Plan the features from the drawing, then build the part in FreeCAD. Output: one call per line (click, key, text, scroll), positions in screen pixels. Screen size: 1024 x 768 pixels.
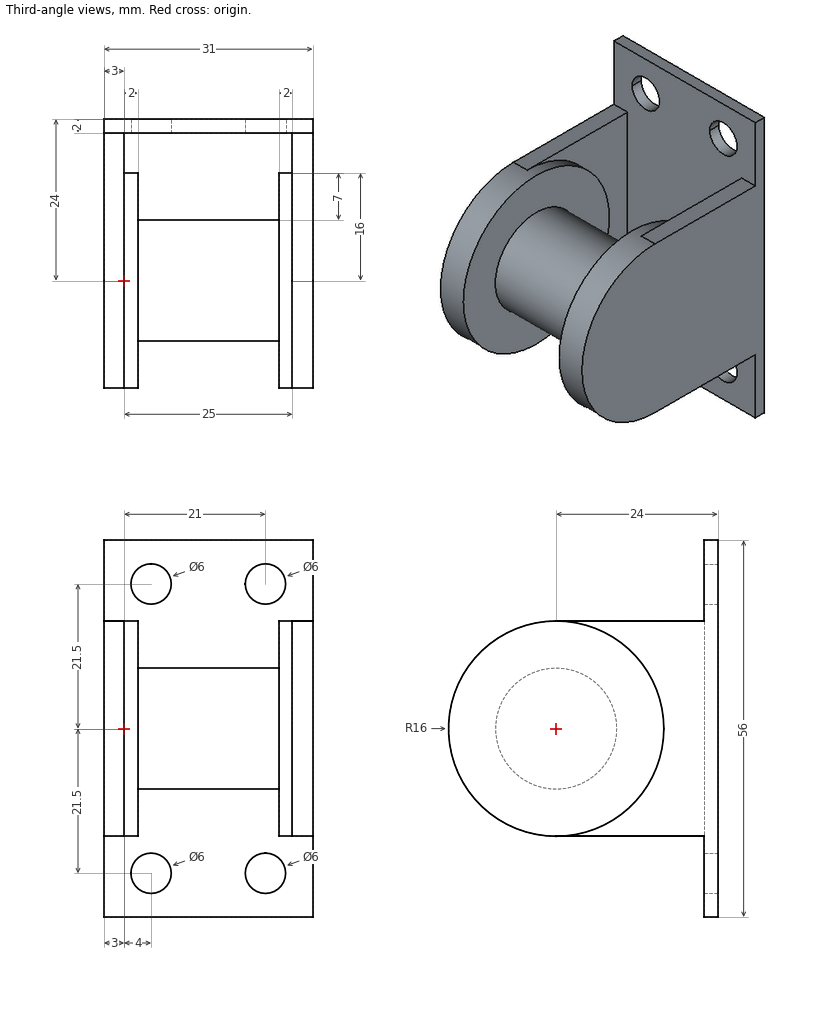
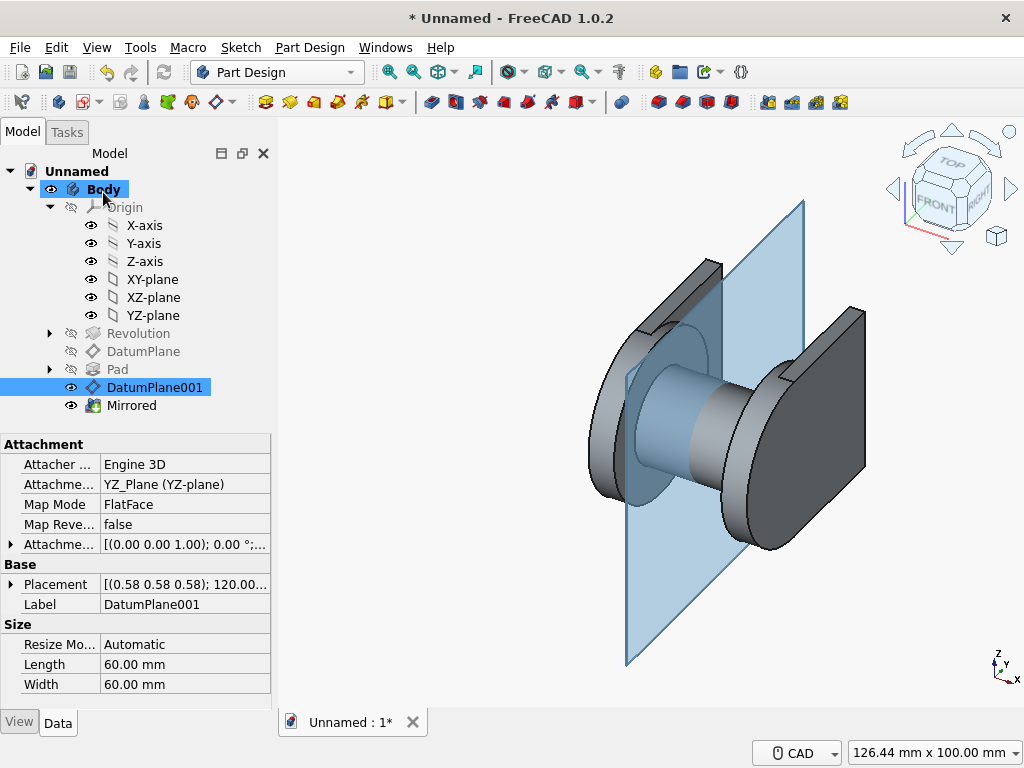
click(116, 387)
key(space)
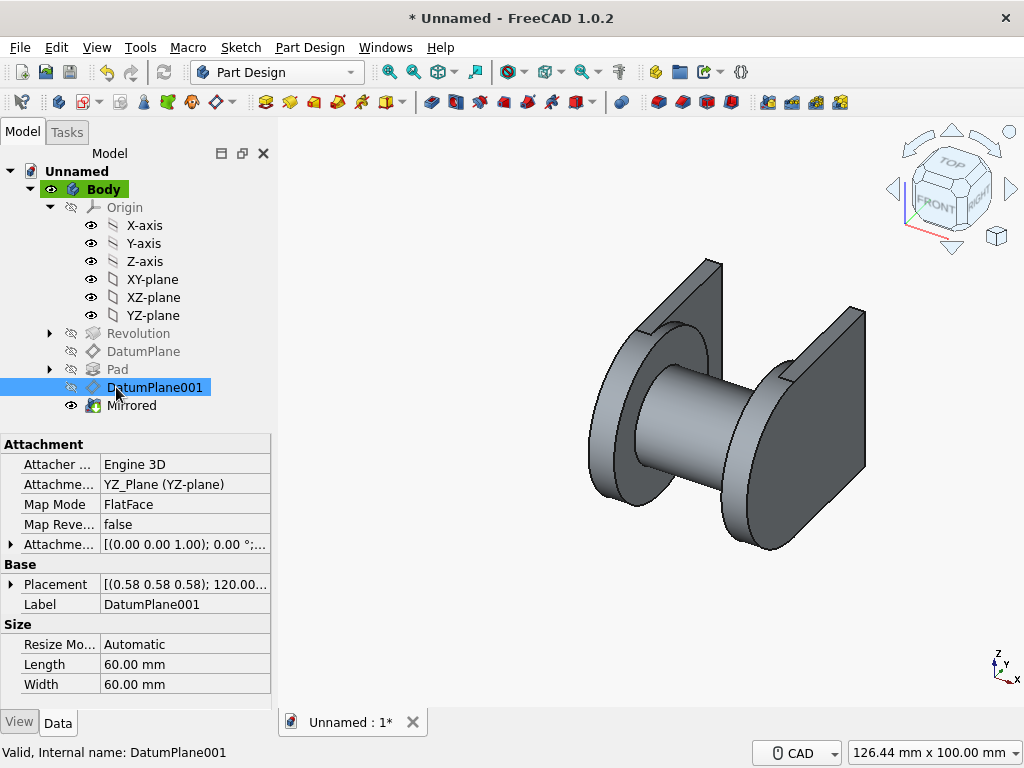
click(318, 667)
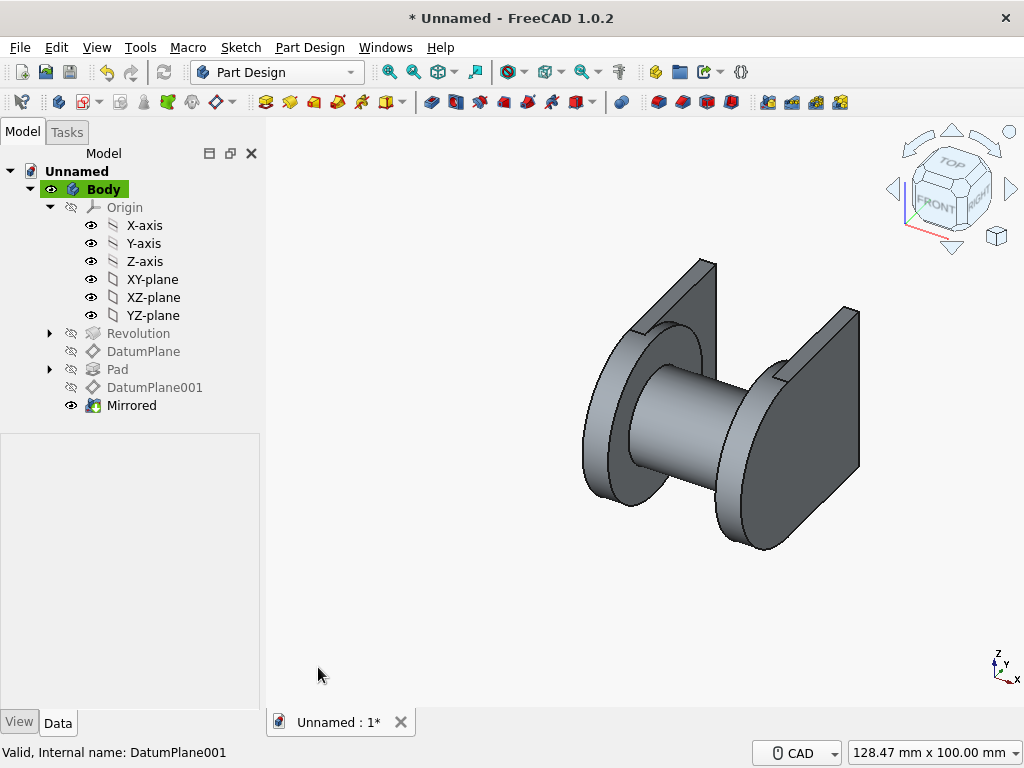
click(84, 102)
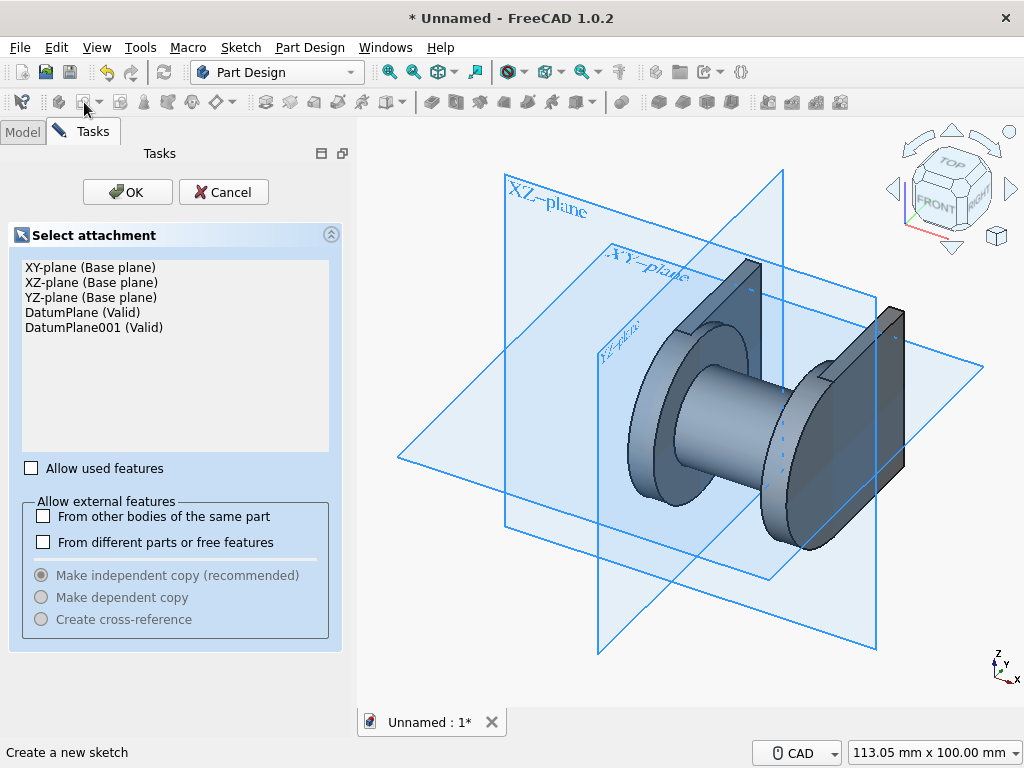
click(82, 268)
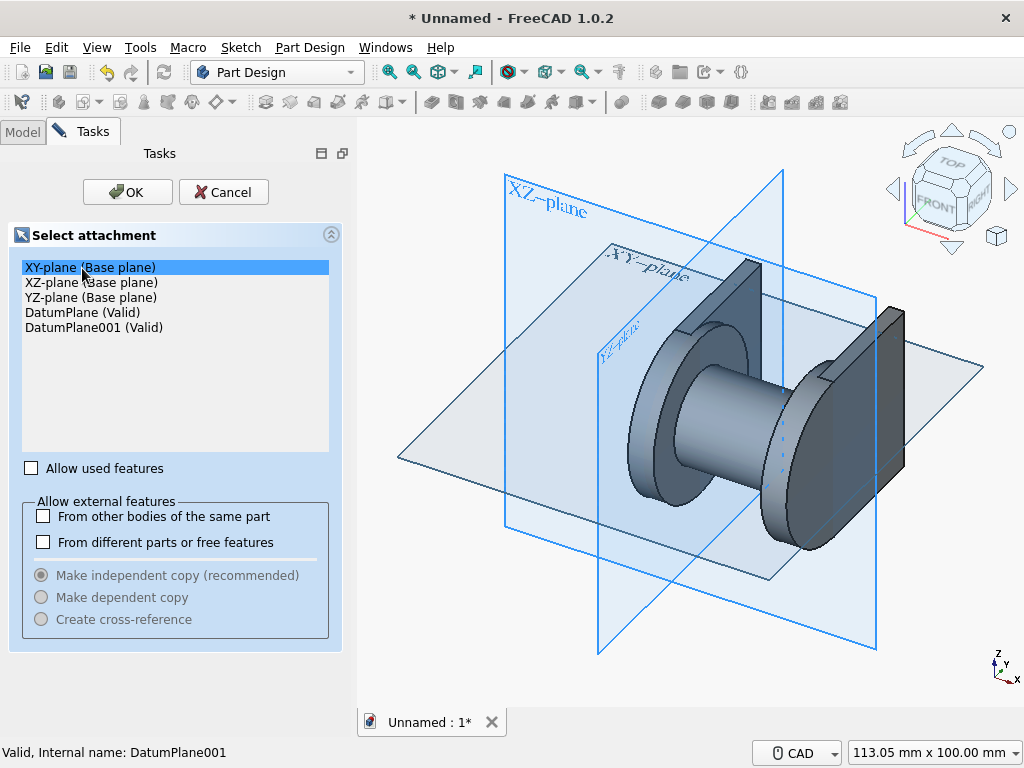
click(128, 192)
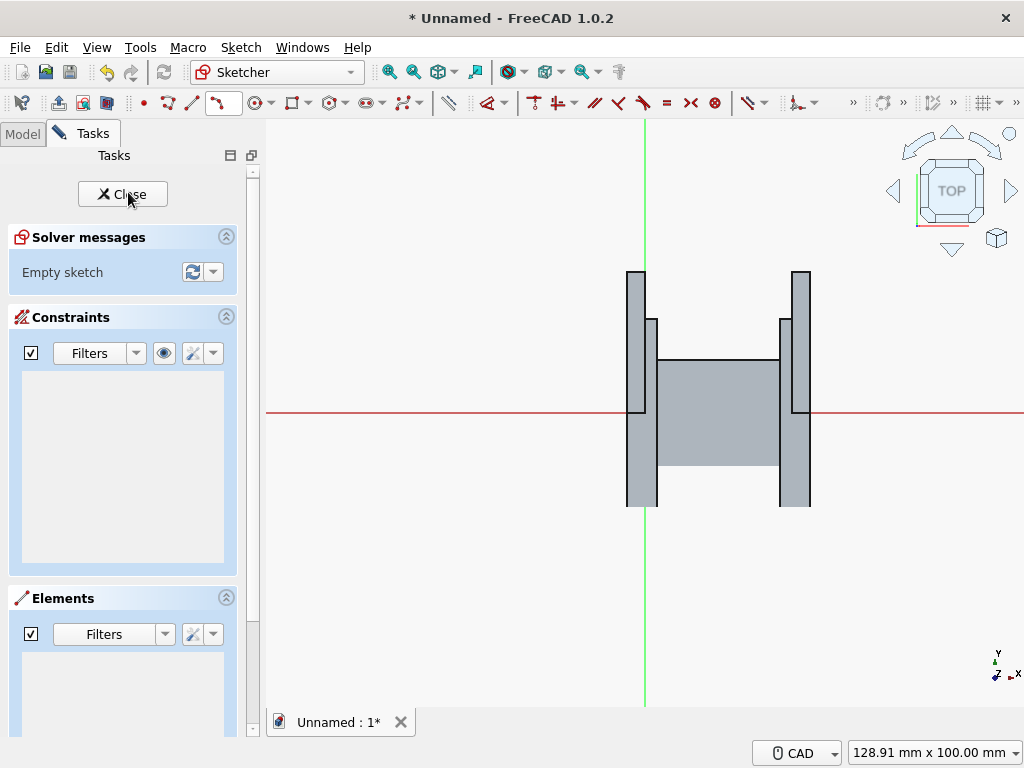
click(108, 104)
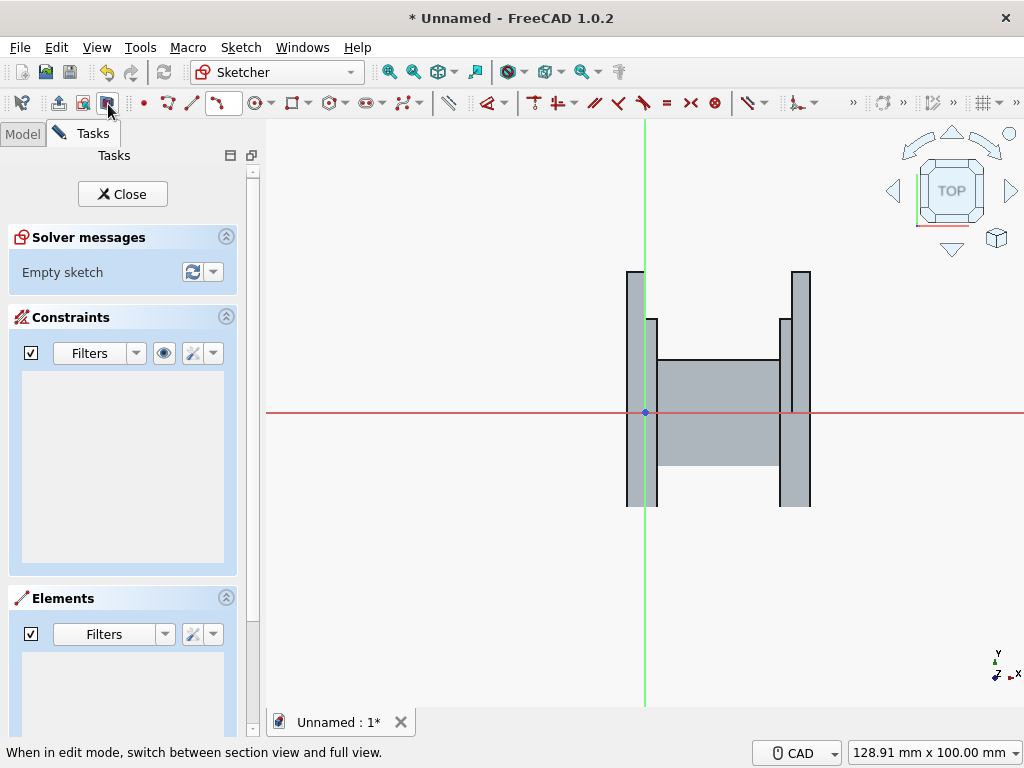
scroll(834, 285, up, 4)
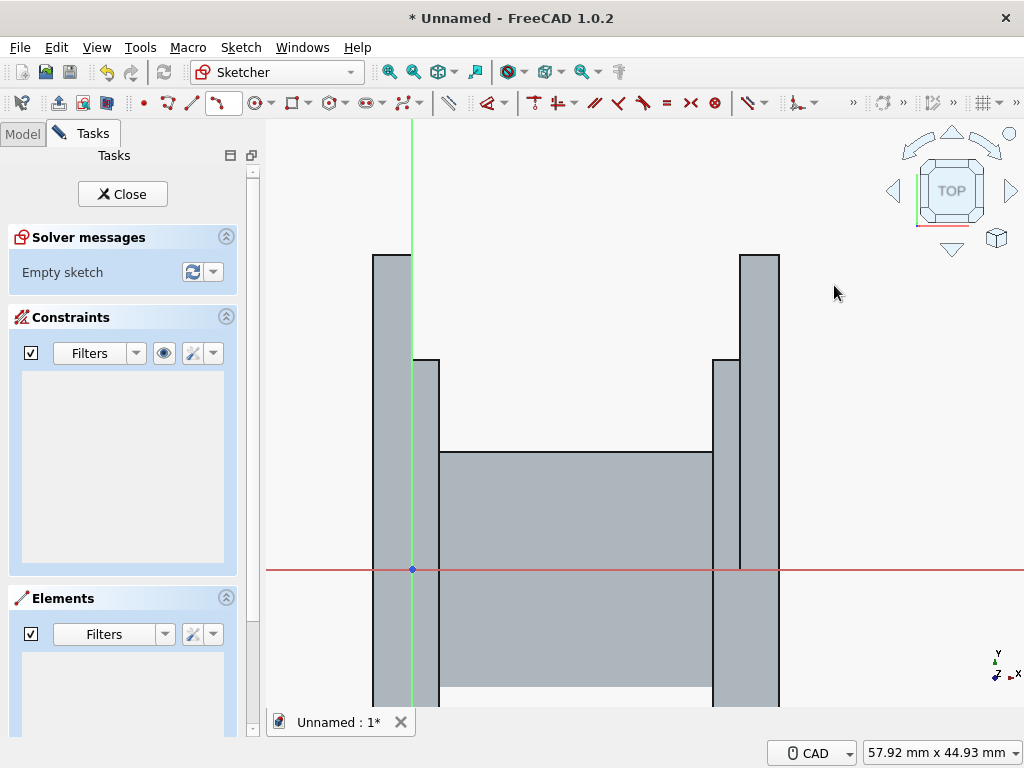
click(292, 104)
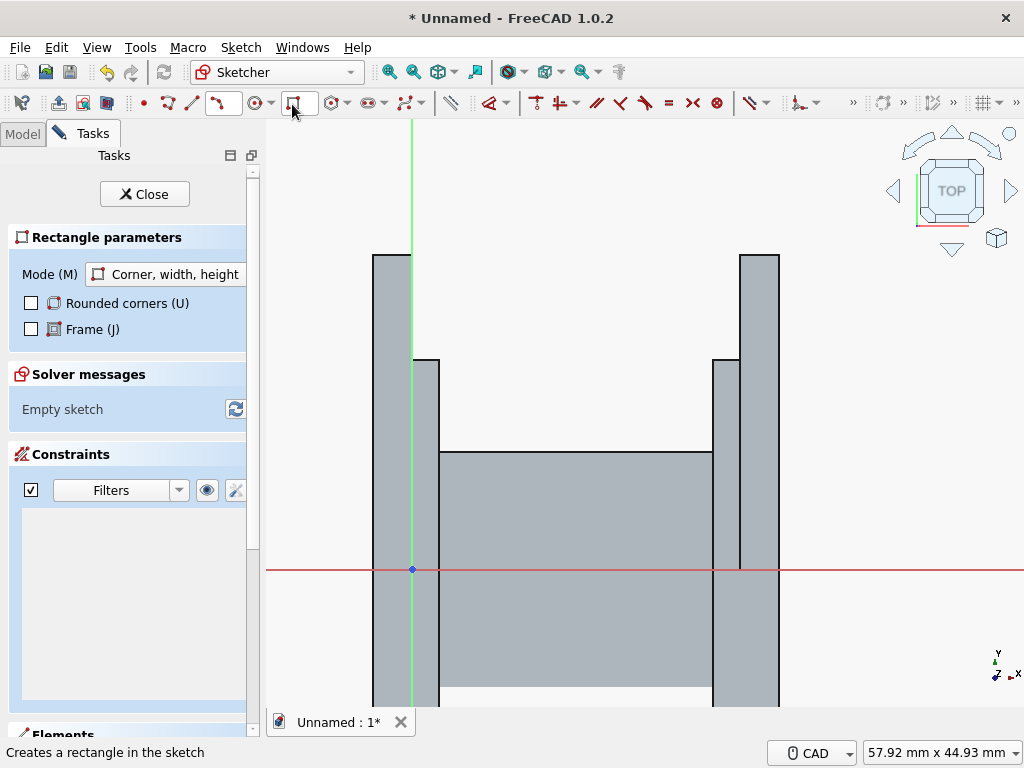
click(373, 255)
click(779, 282)
key(Escape)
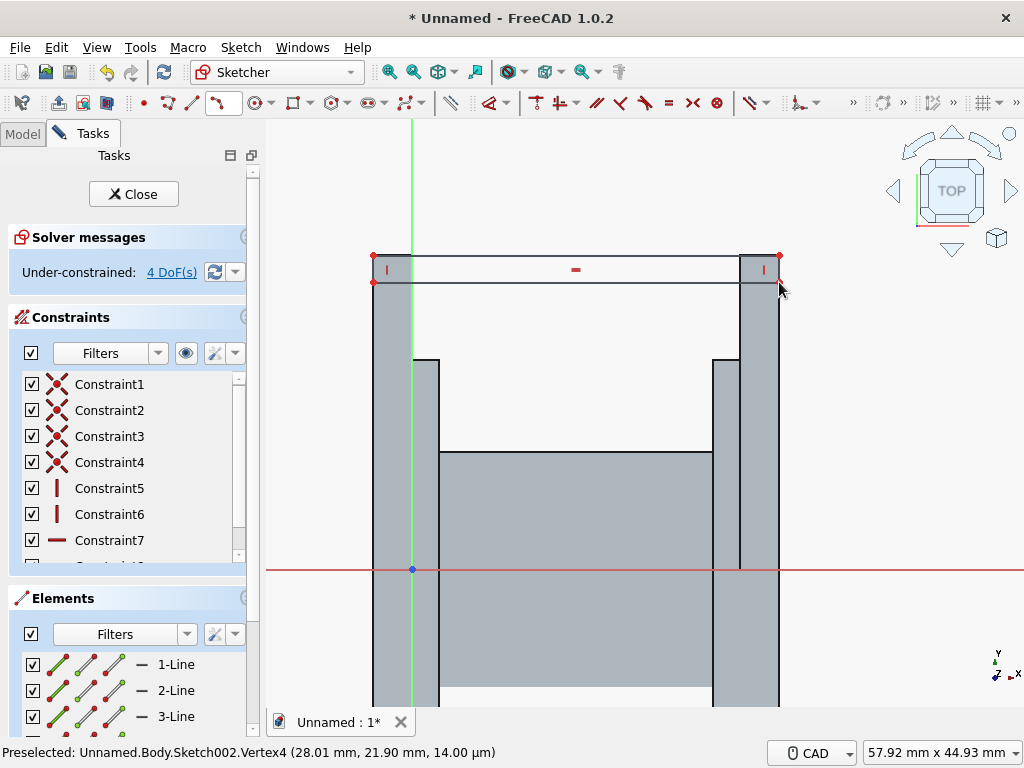
click(490, 104)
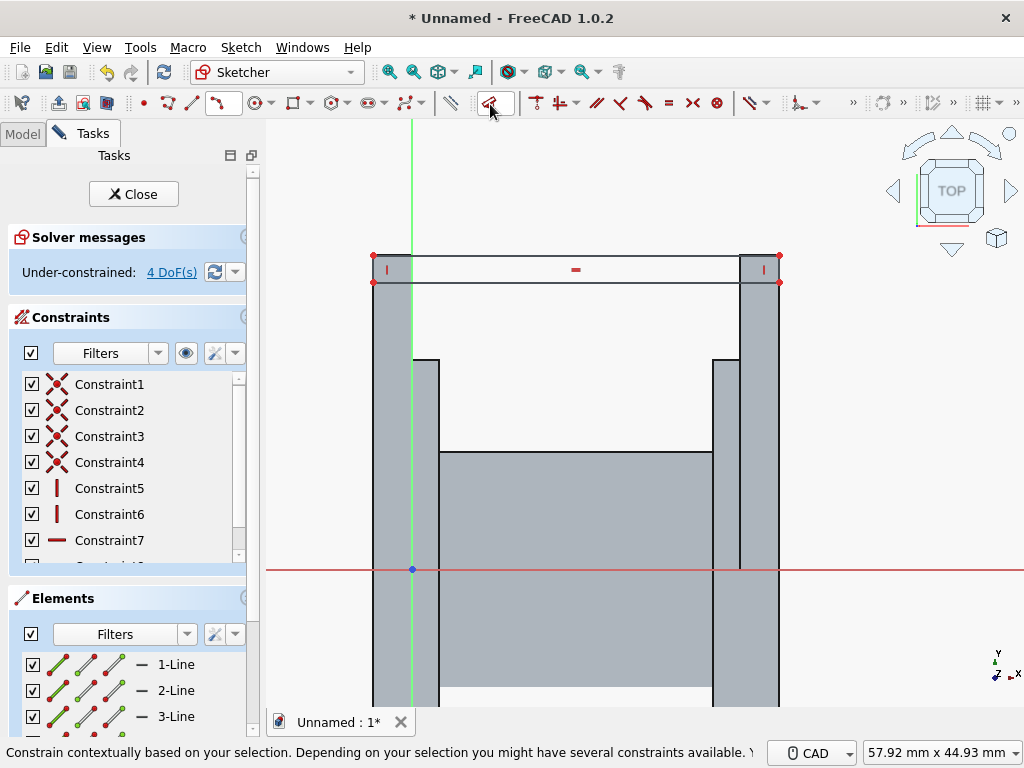
scroll(373, 267, up, 3)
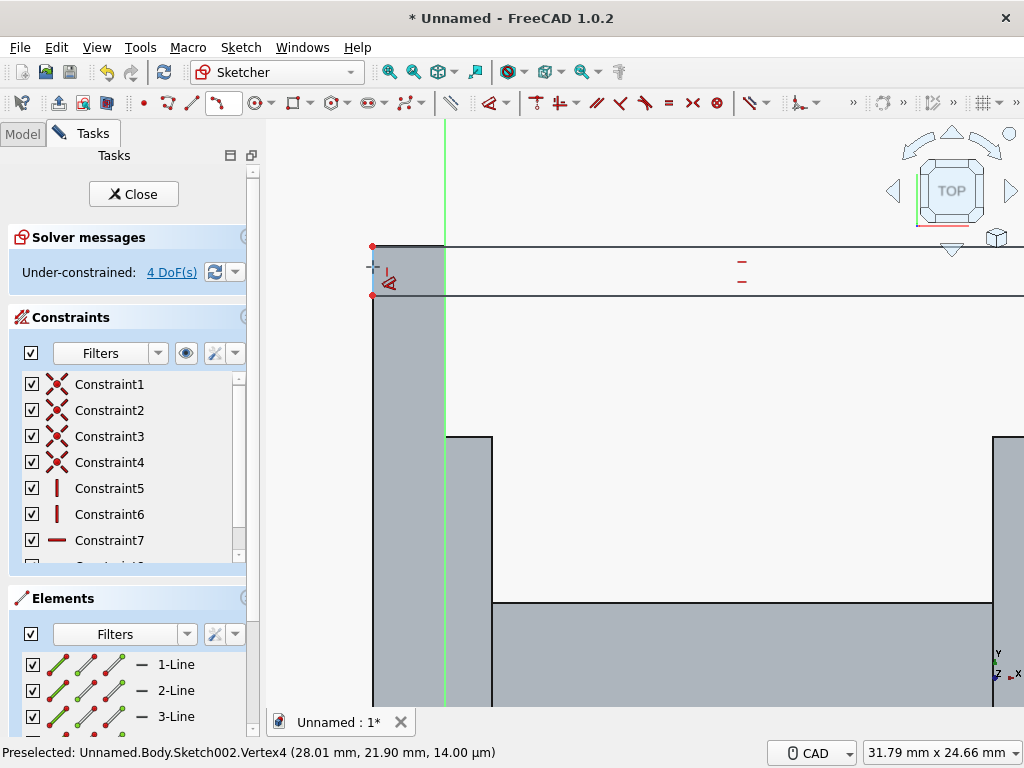
click(373, 266)
click(339, 271)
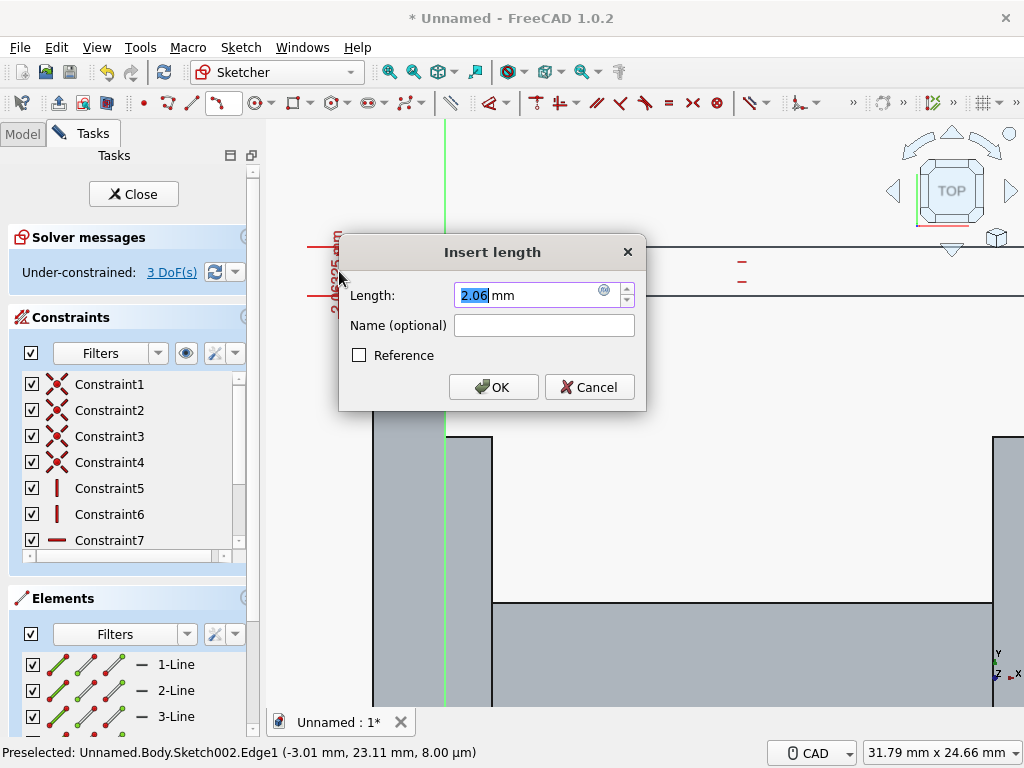
text(2)
key(Return)